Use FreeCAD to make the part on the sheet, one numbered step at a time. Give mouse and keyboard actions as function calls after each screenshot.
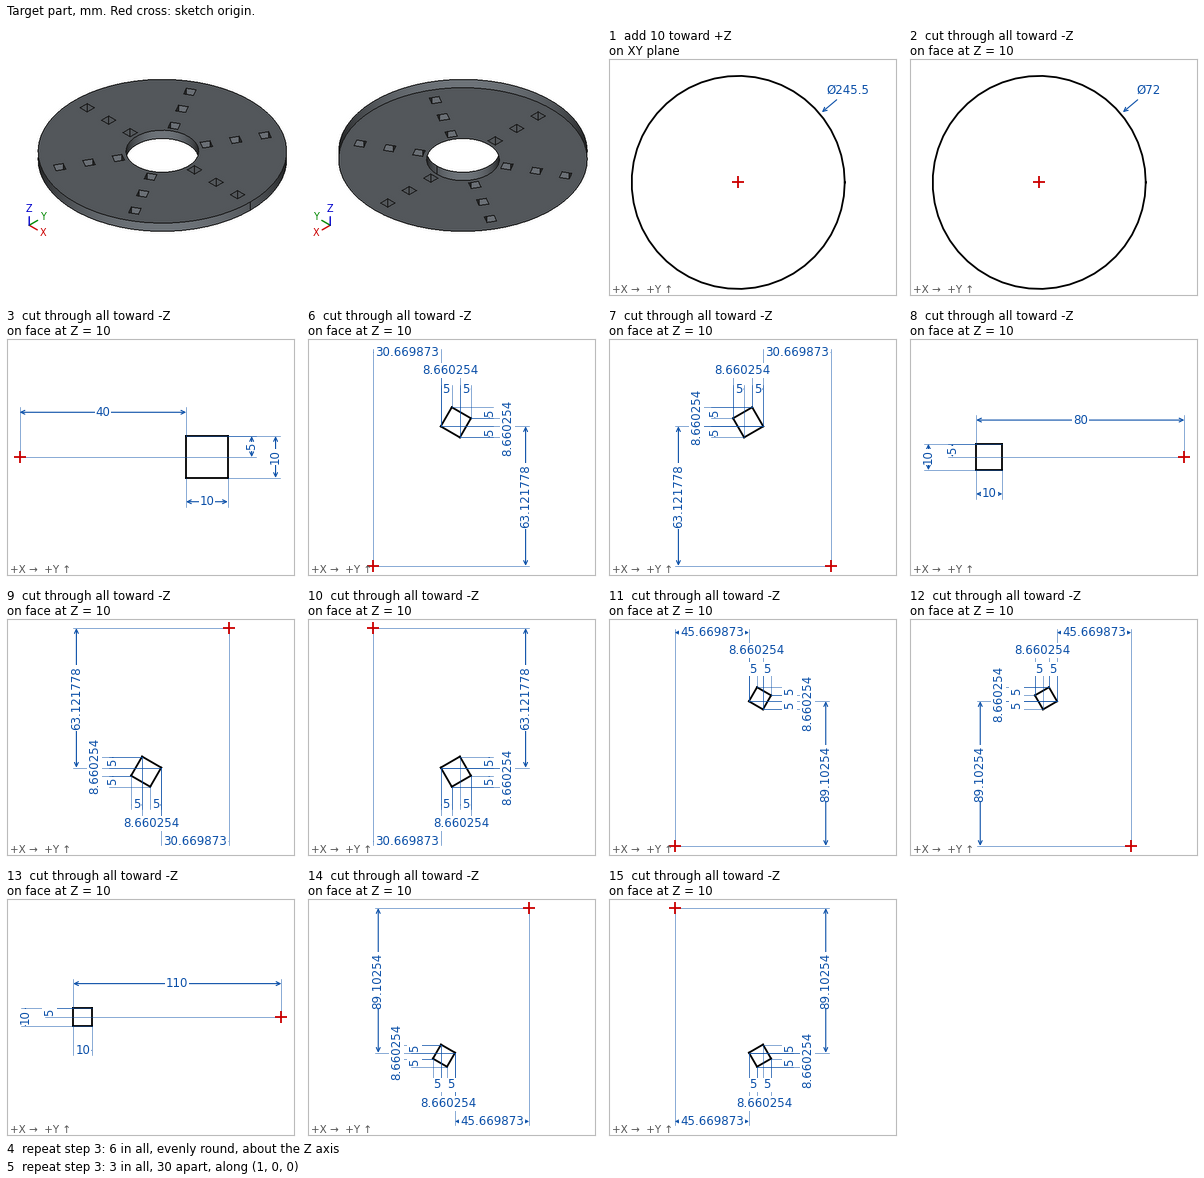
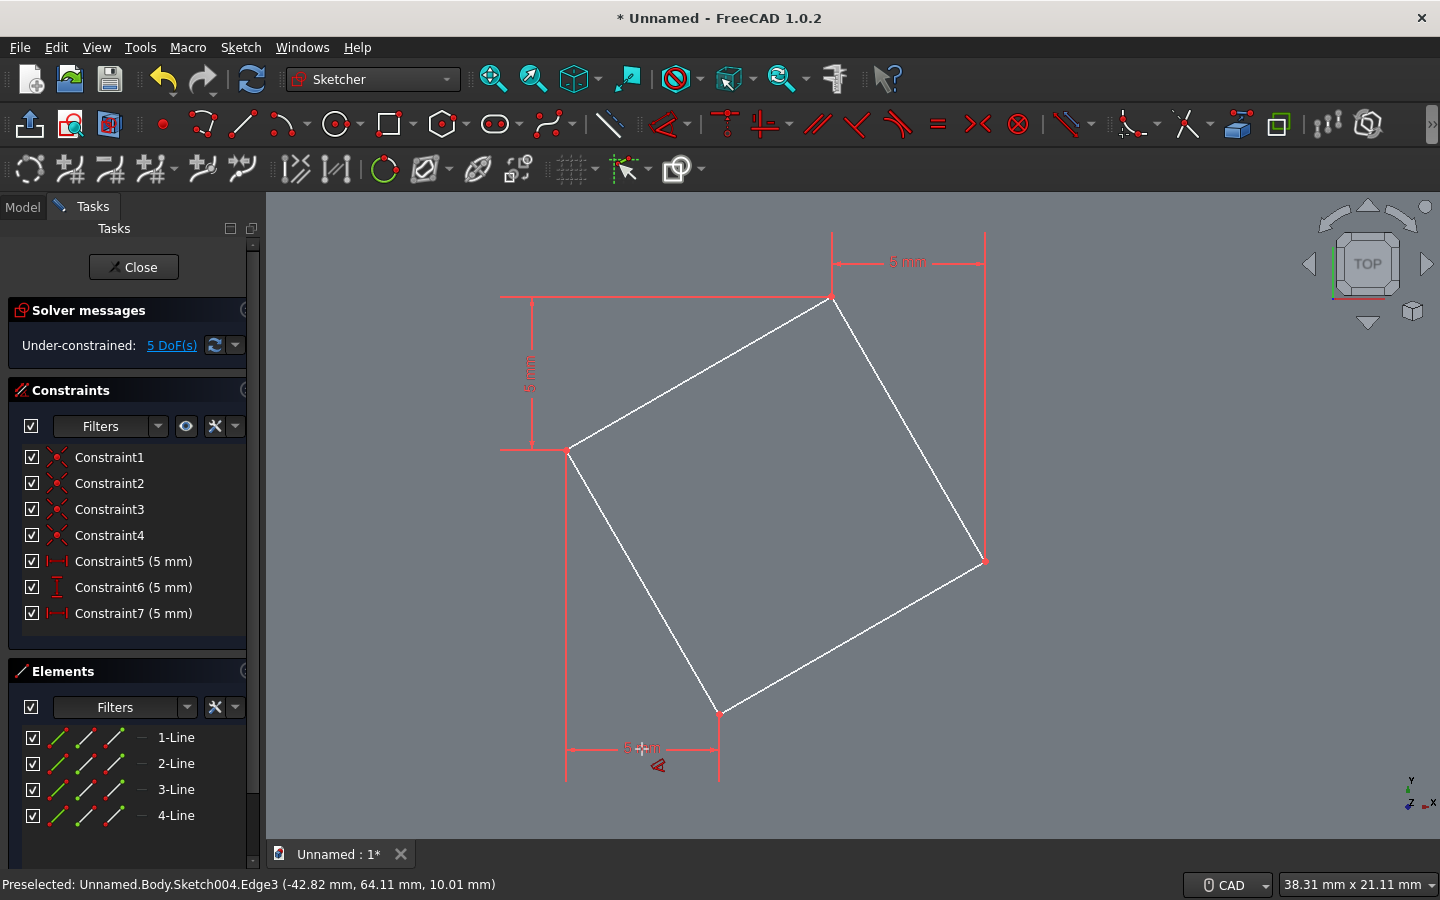
click(799, 669)
click(1019, 639)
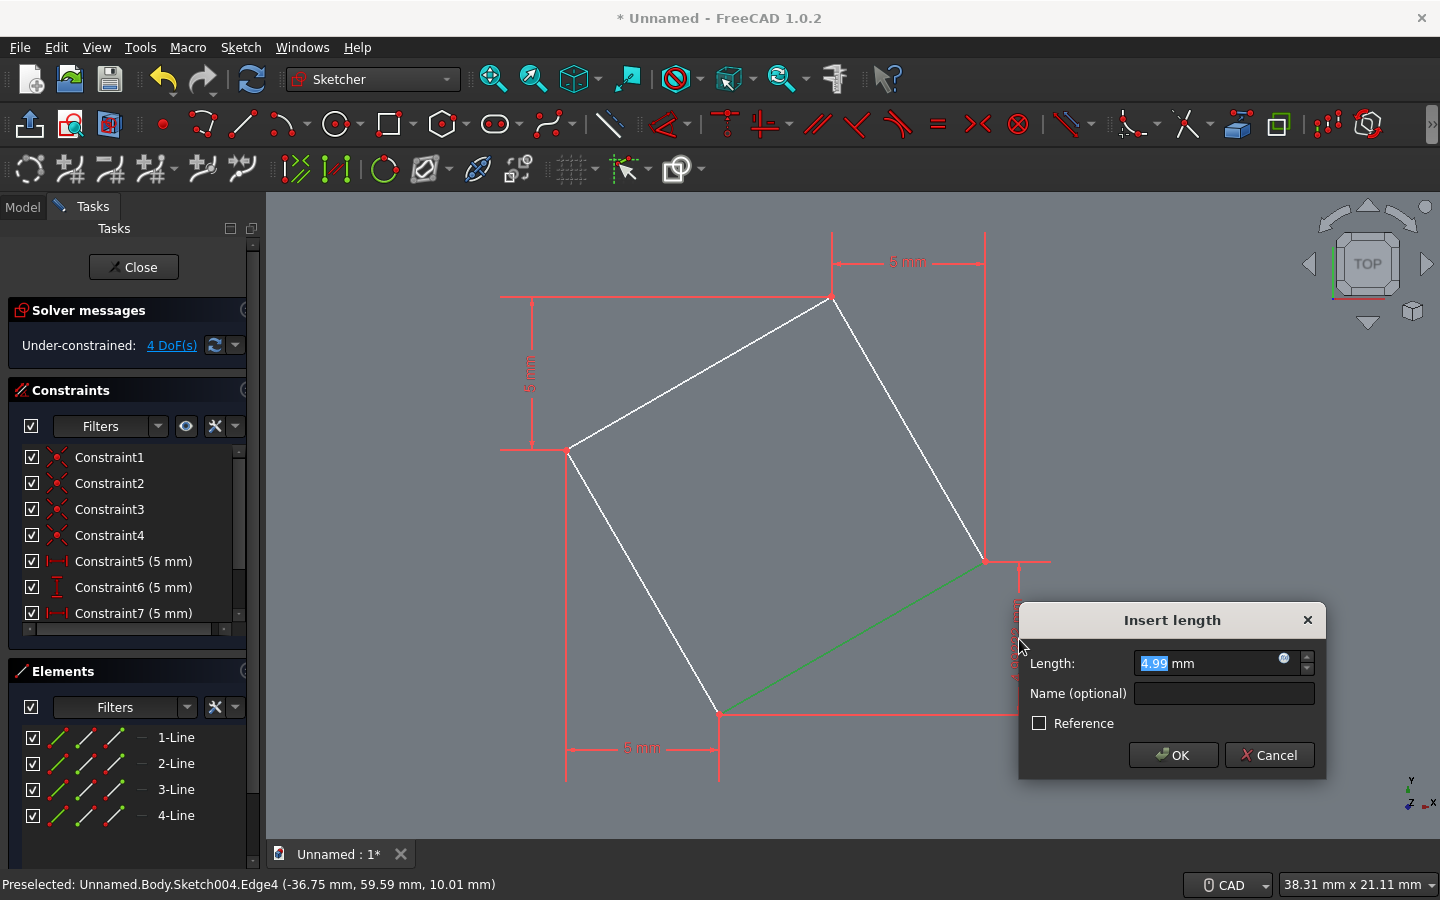
text(5)
key(Return)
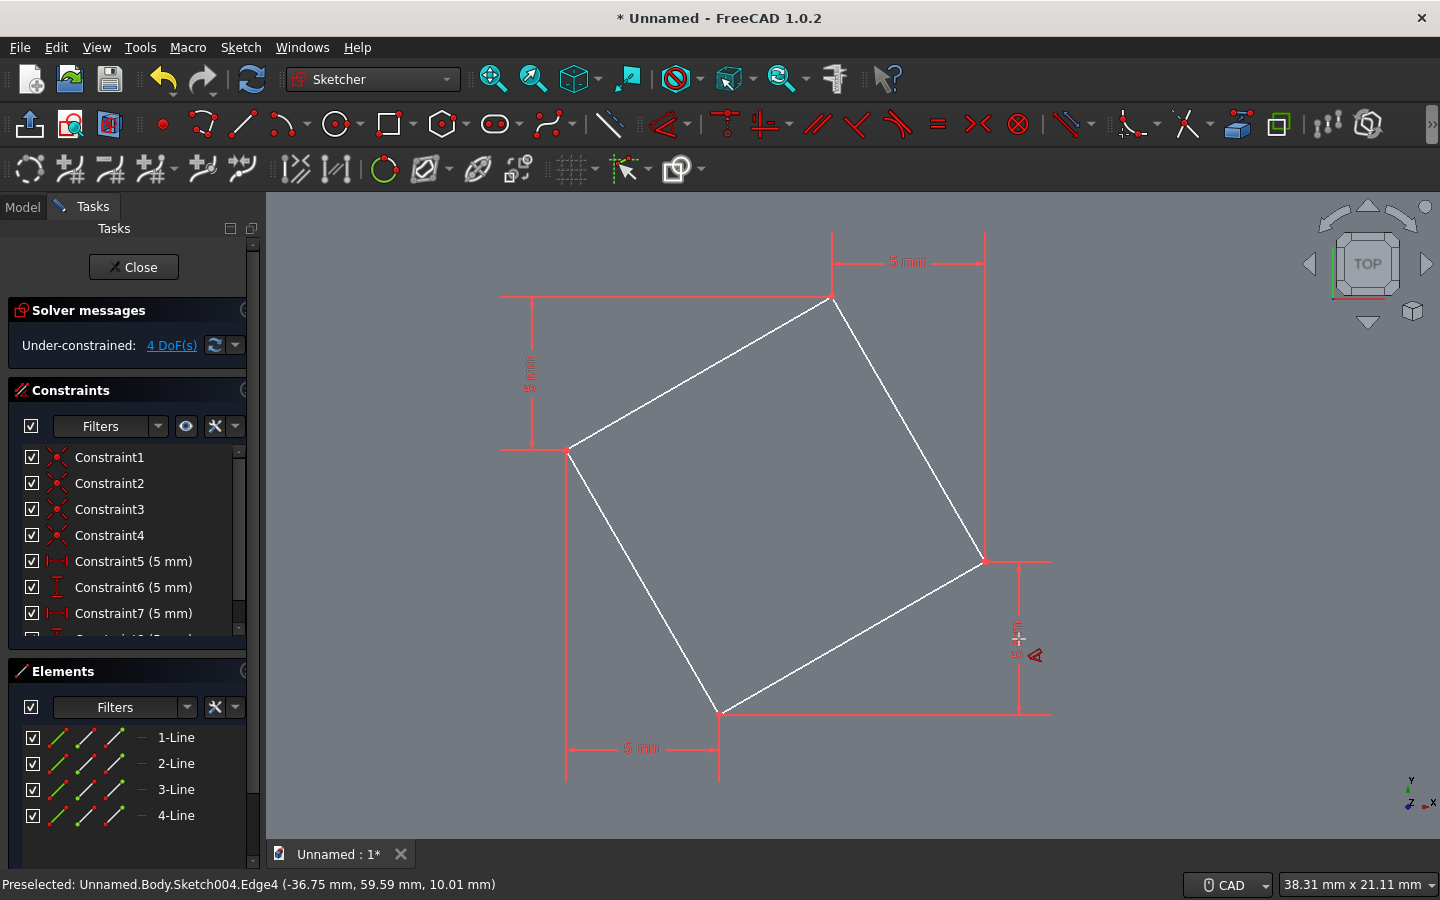
click(939, 482)
click(1019, 429)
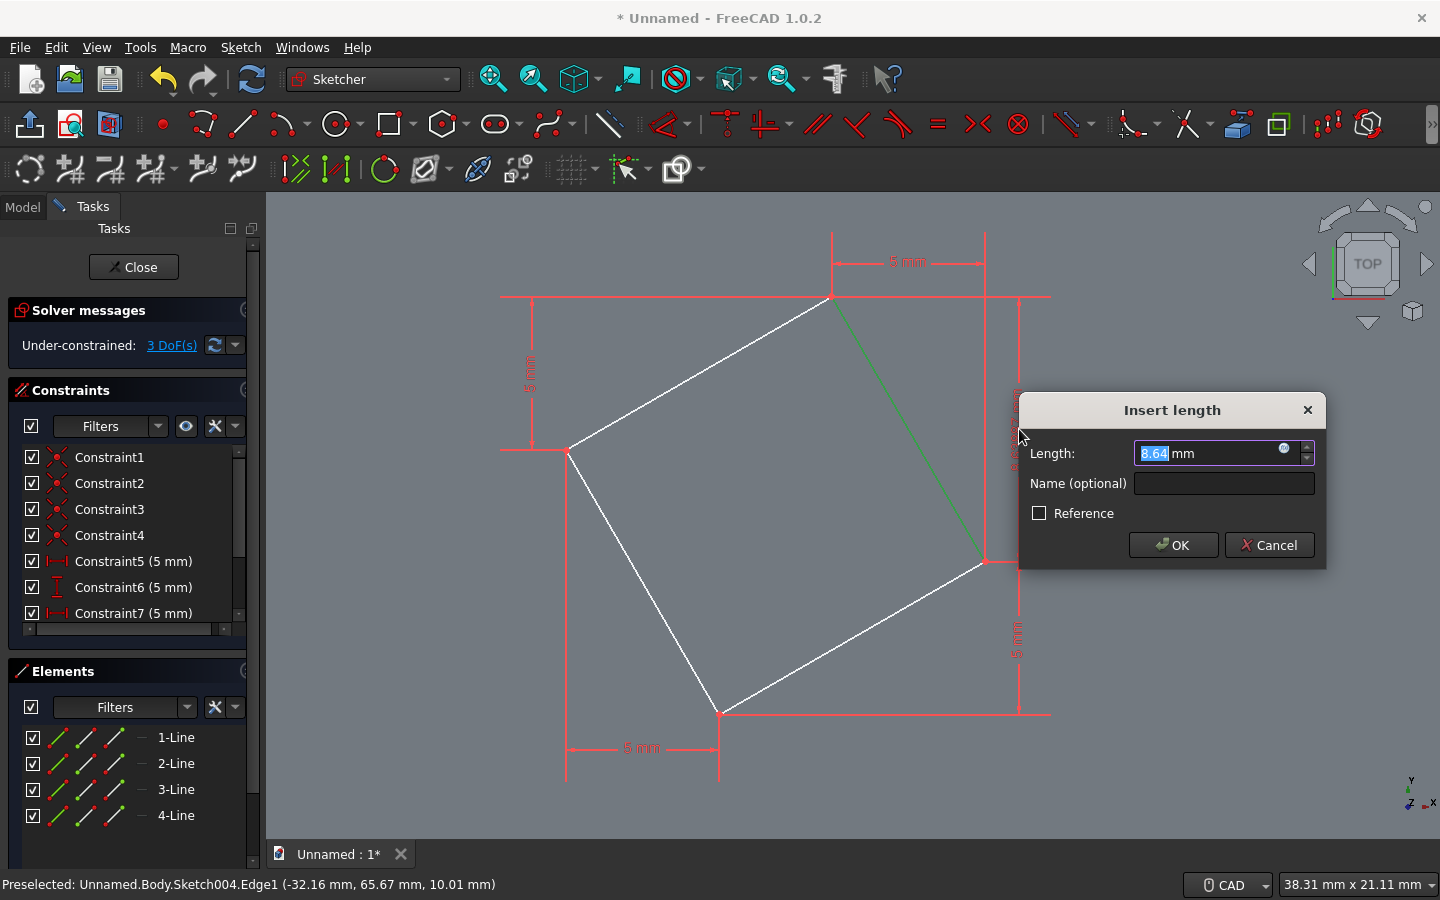
text(8.660254)
key(Return)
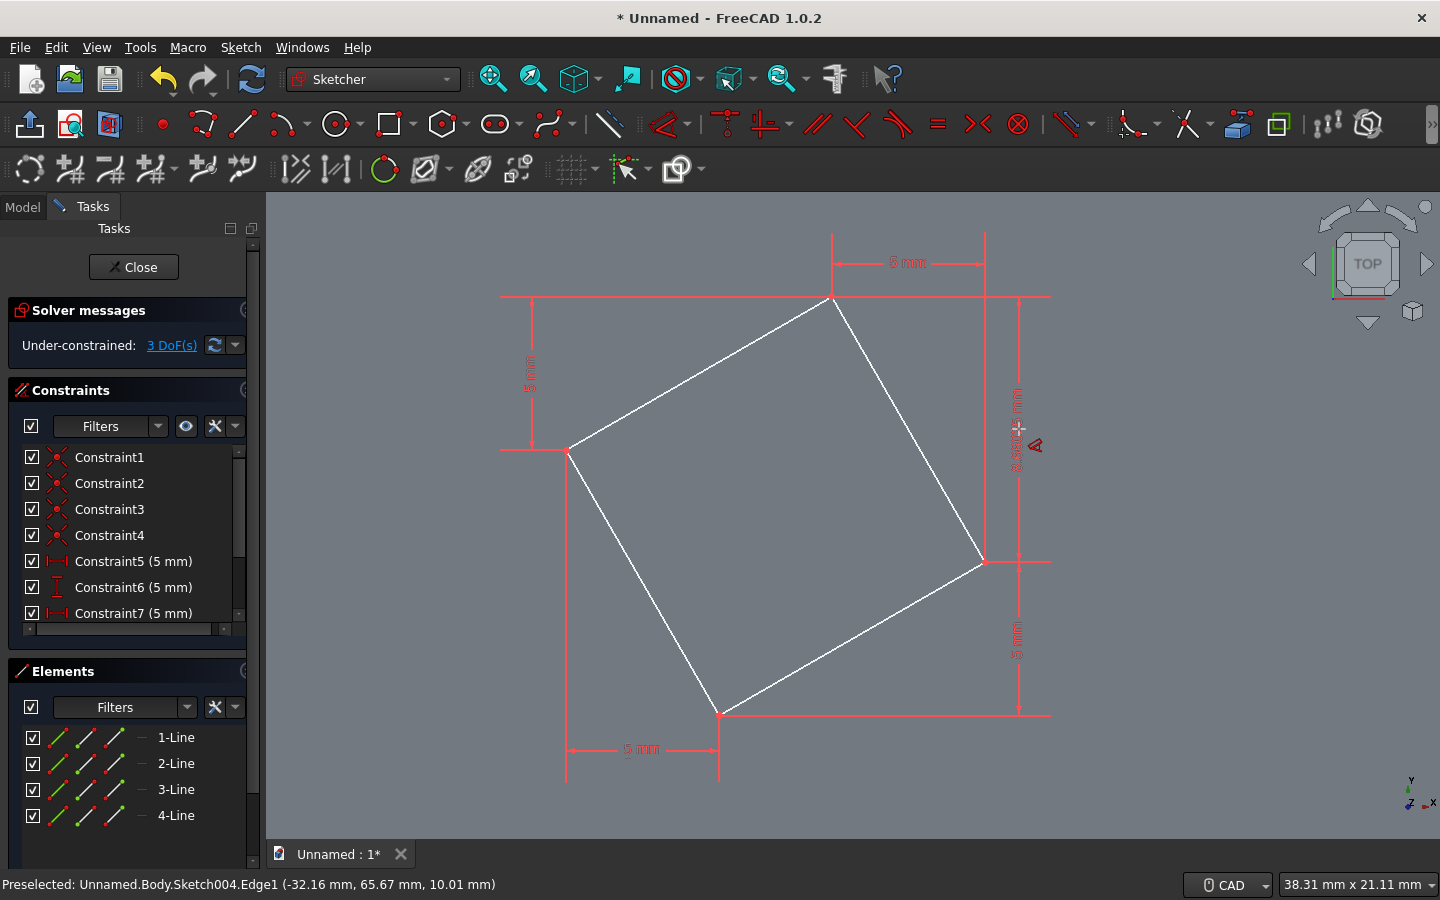
click(752, 343)
click(699, 263)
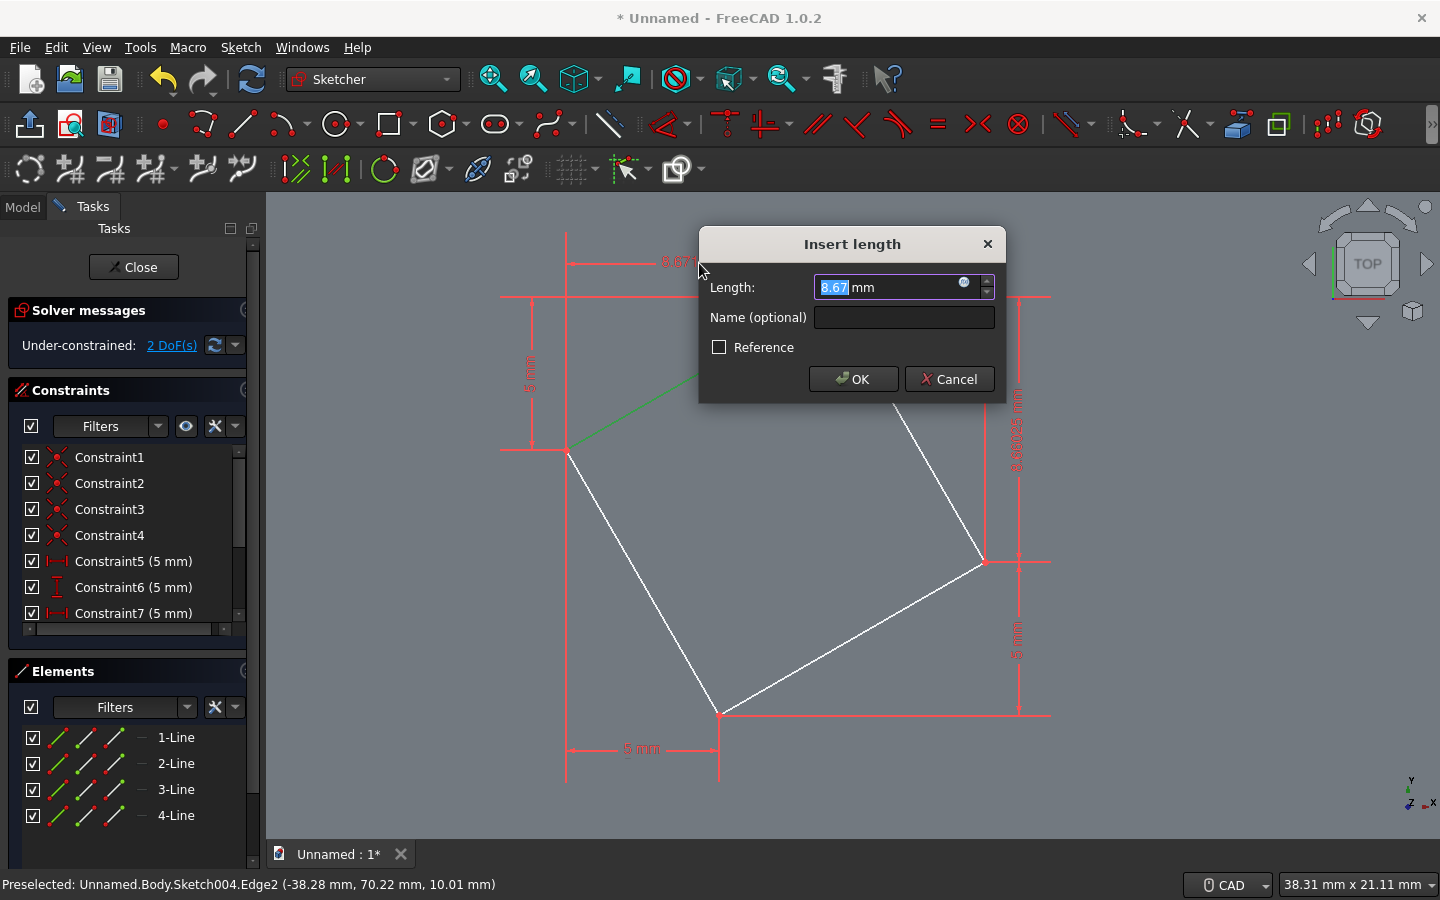
text(8.660254)
key(Return)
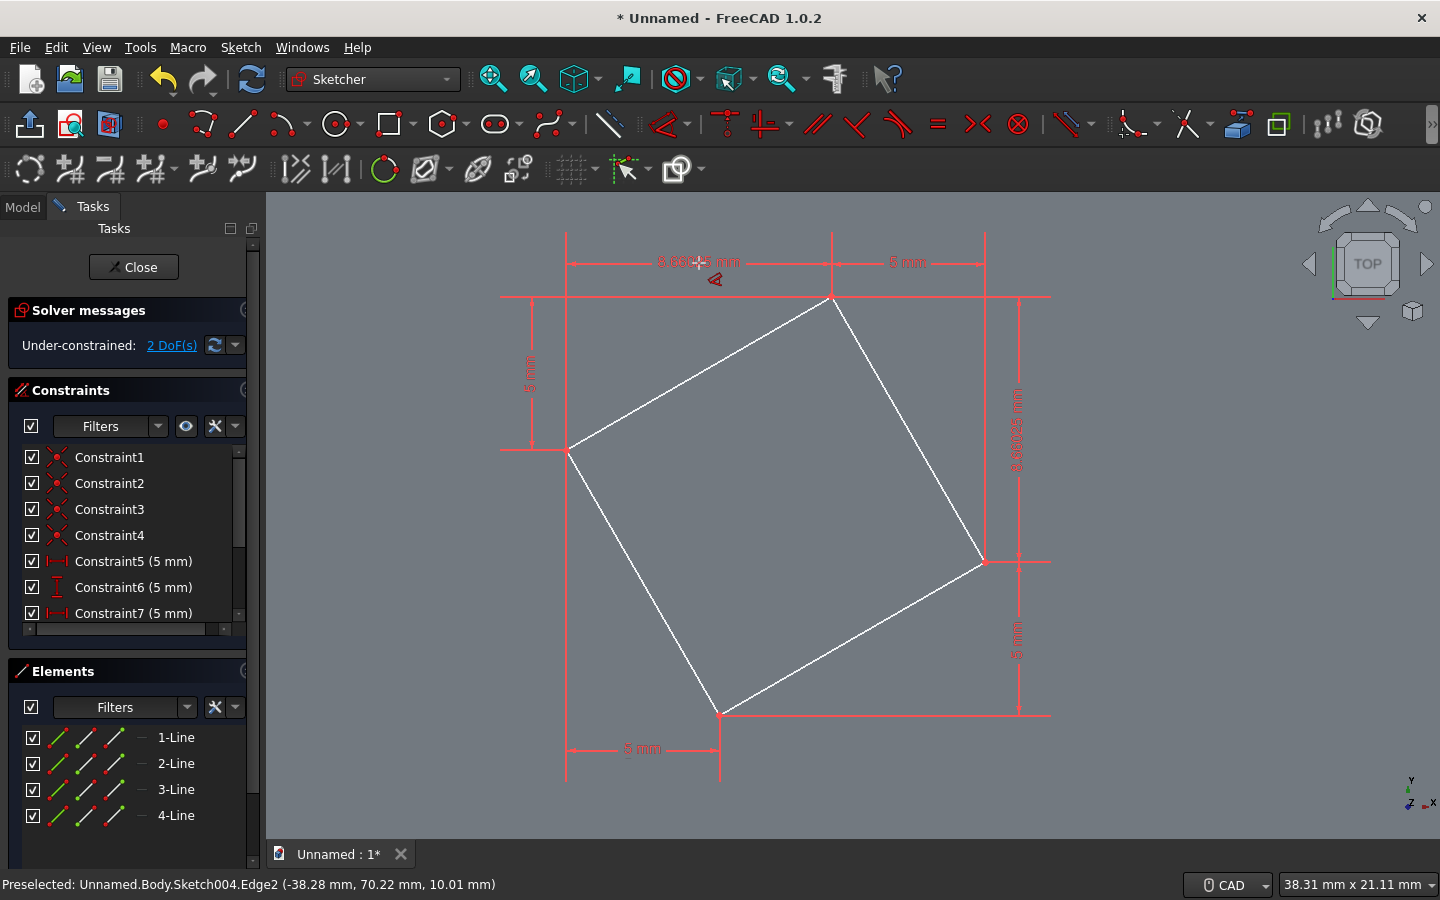
click(985, 562)
click(1130, 528)